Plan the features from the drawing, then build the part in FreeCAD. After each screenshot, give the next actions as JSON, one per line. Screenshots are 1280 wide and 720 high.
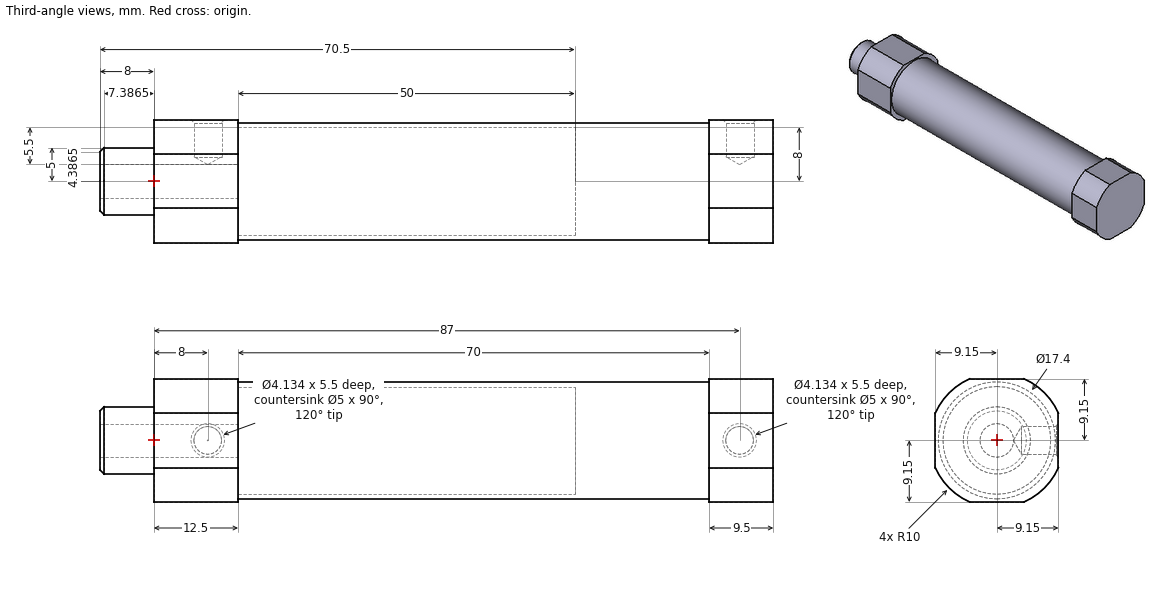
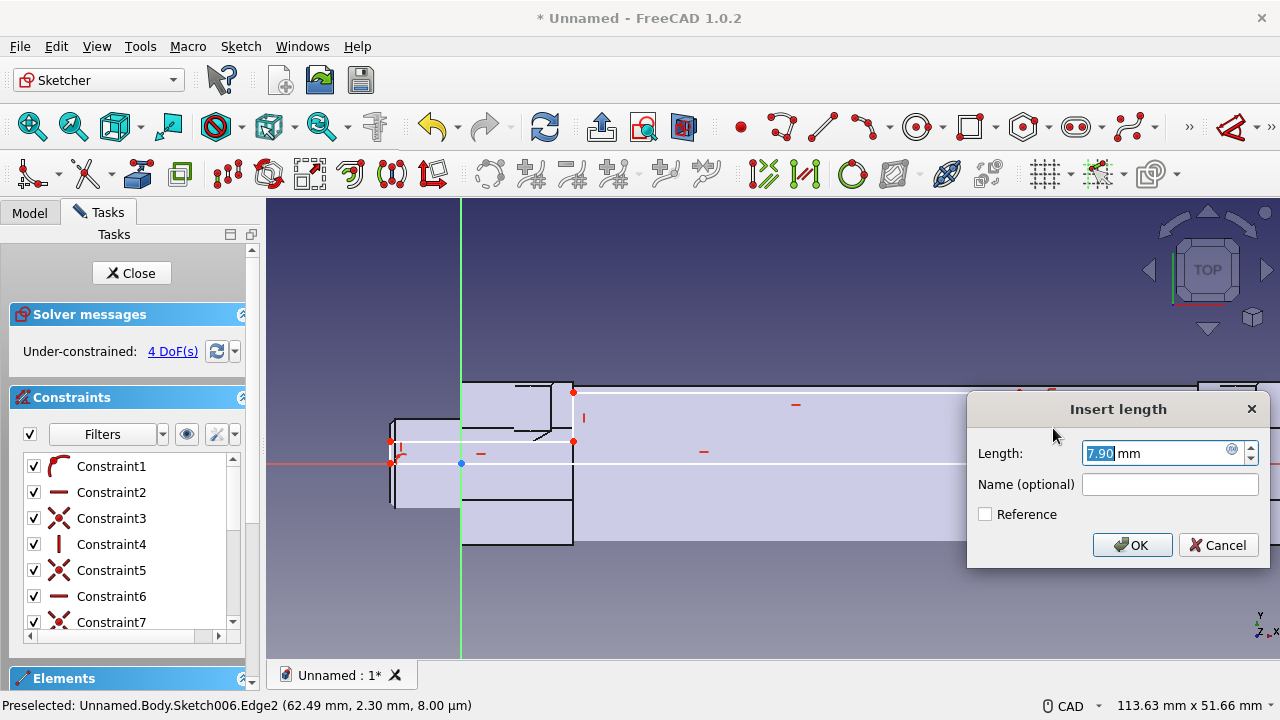
{"action": "type", "text": "8"}
{"action": "key", "text": "Return"}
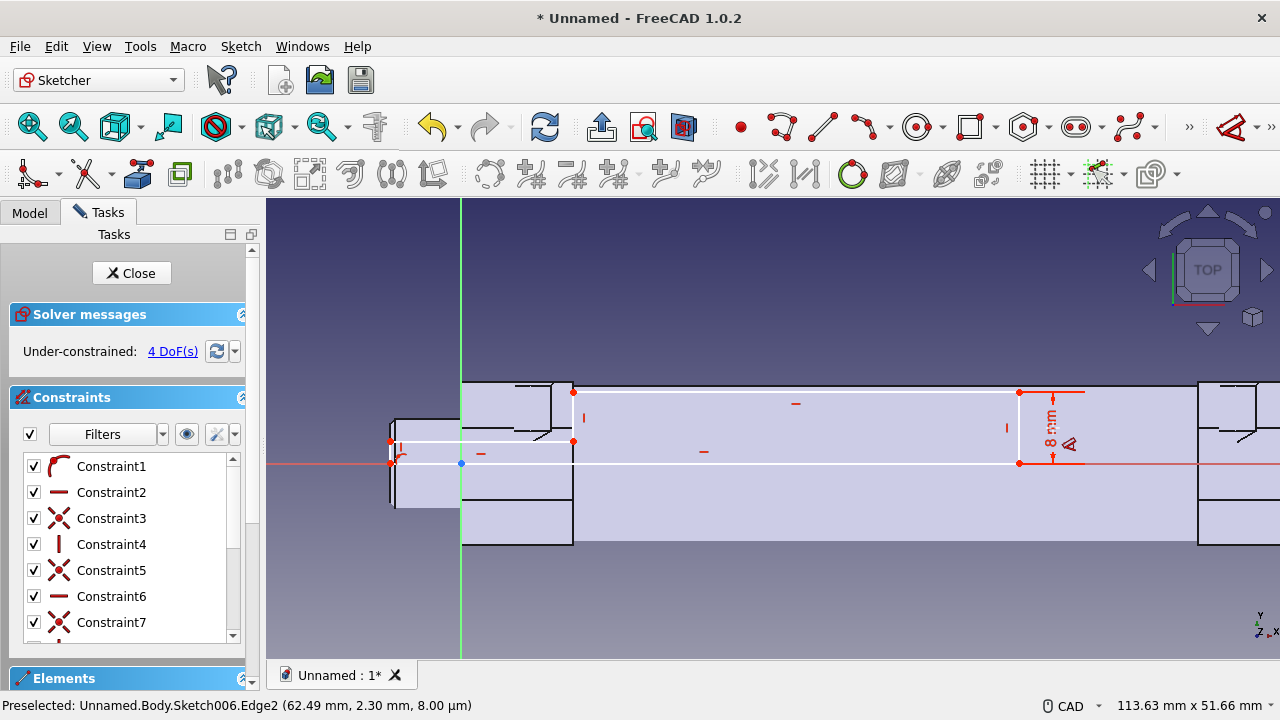
{"action": "left_click", "coordinate": [885, 392]}
{"action": "left_click", "coordinate": [796, 358]}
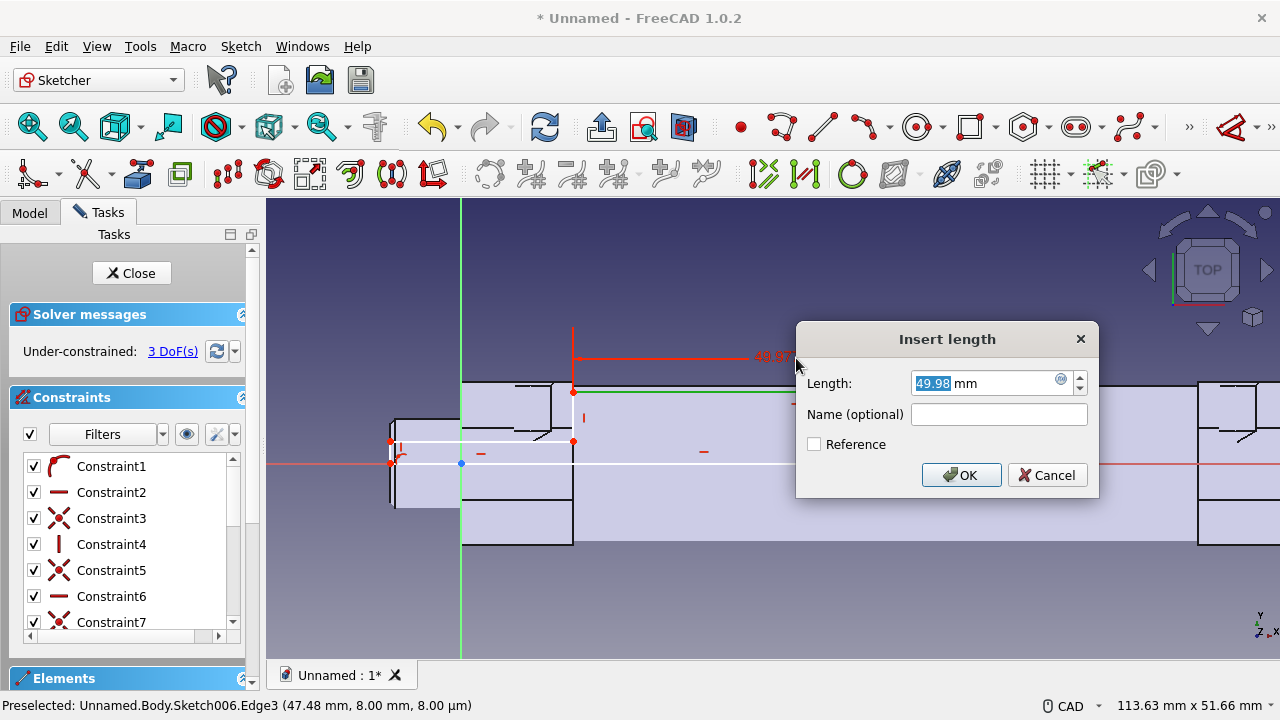
{"action": "type", "text": "50"}
{"action": "key", "text": "Return"}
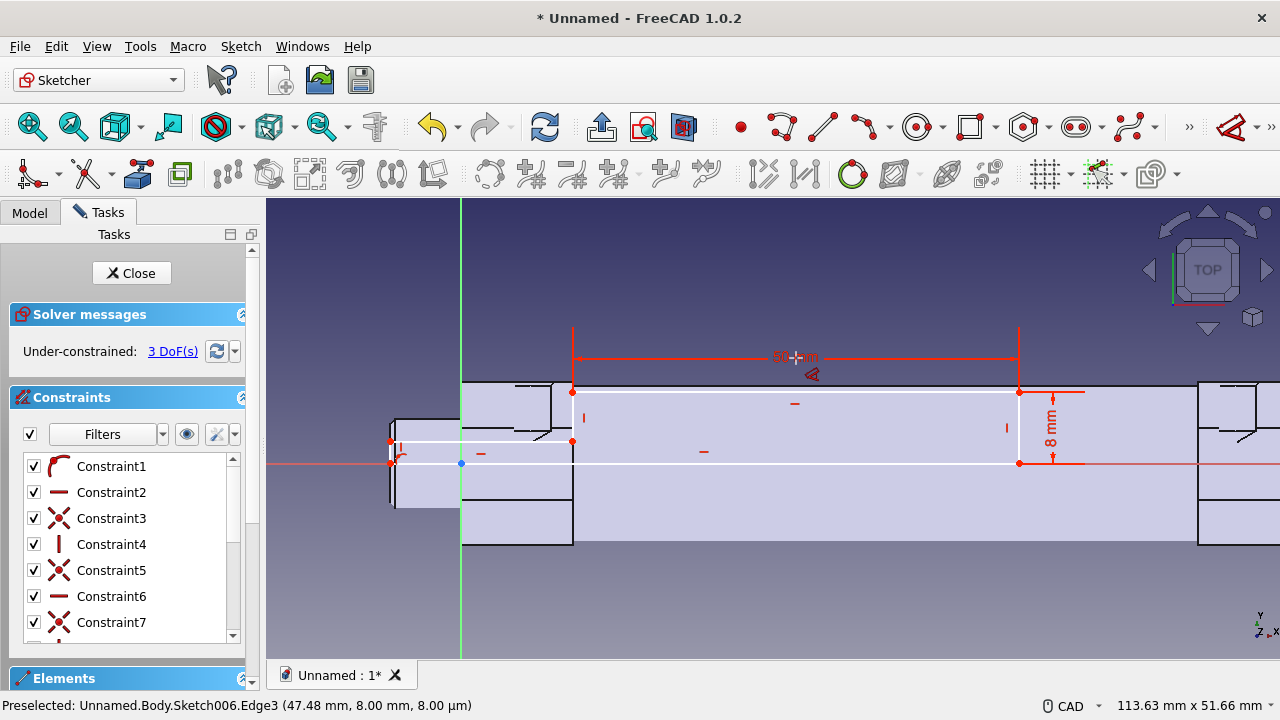
{"action": "left_click", "coordinate": [390, 464]}
{"action": "left_click", "coordinate": [426, 498]}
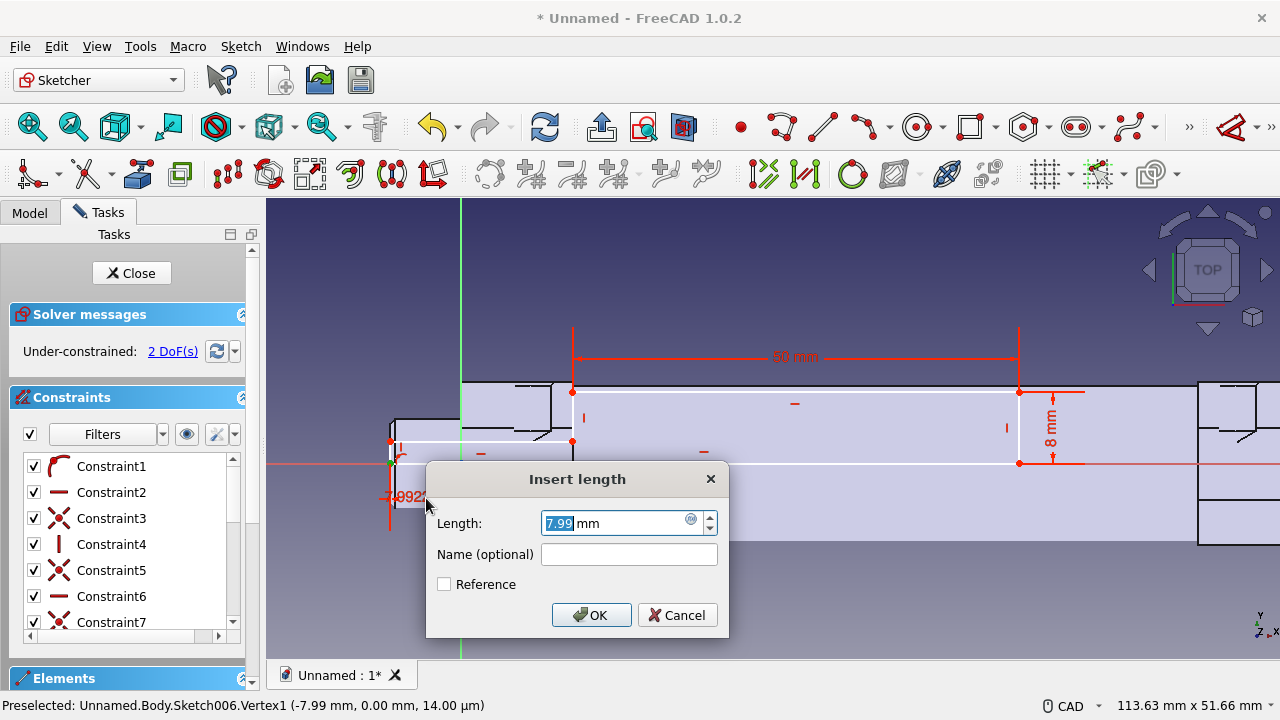
{"action": "type", "text": "8"}
{"action": "key", "text": "Return"}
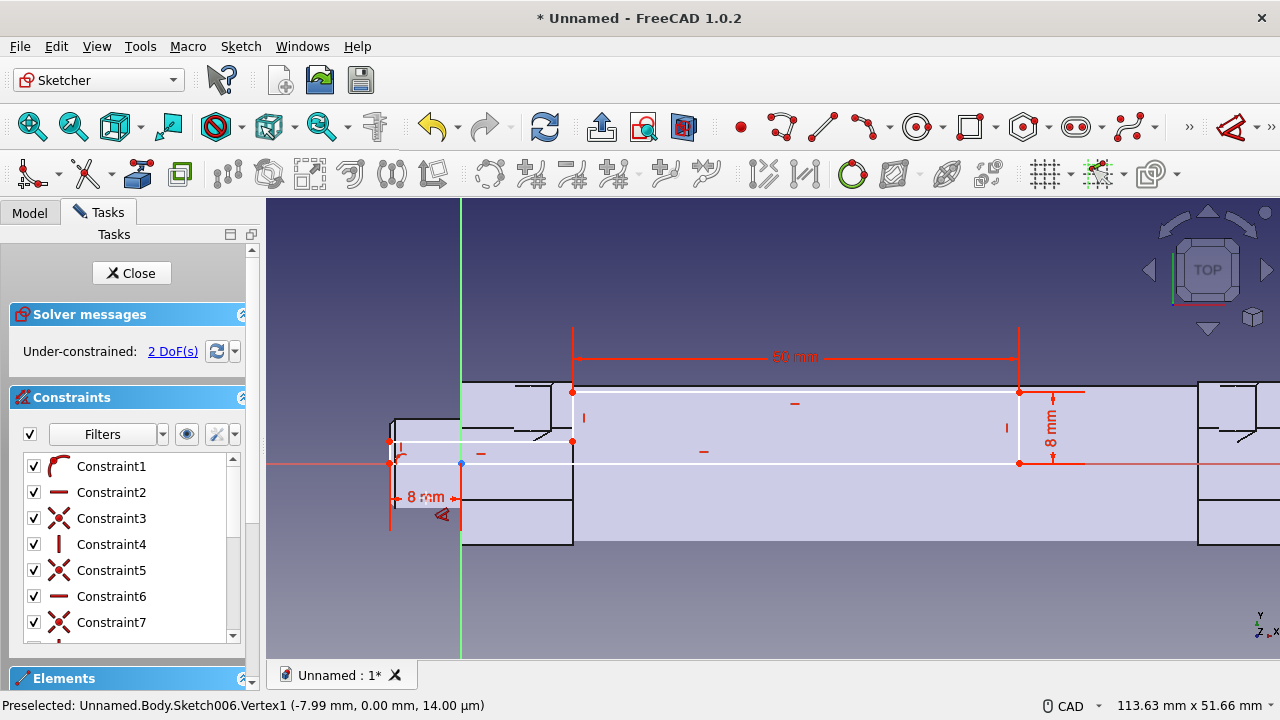
{"action": "left_click", "coordinate": [573, 407]}
{"action": "left_click", "coordinate": [539, 417]}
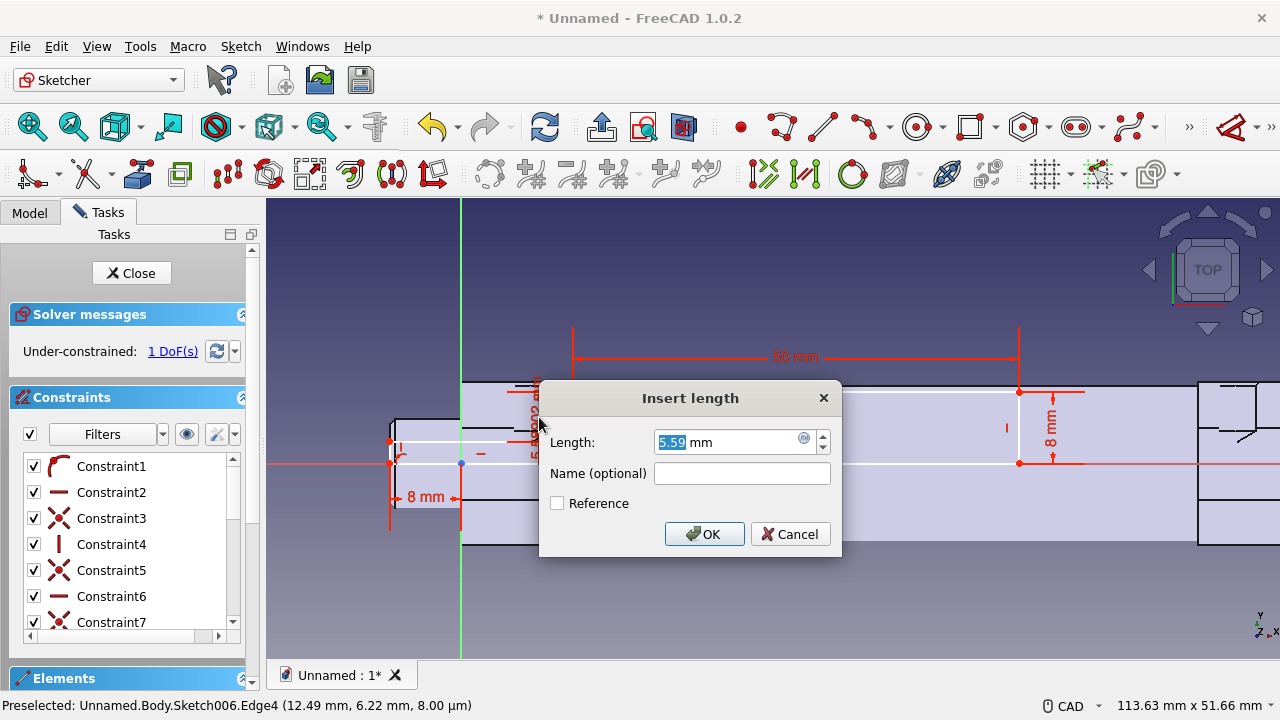
{"action": "type", "text": "5.5"}
{"action": "key", "text": "Return"}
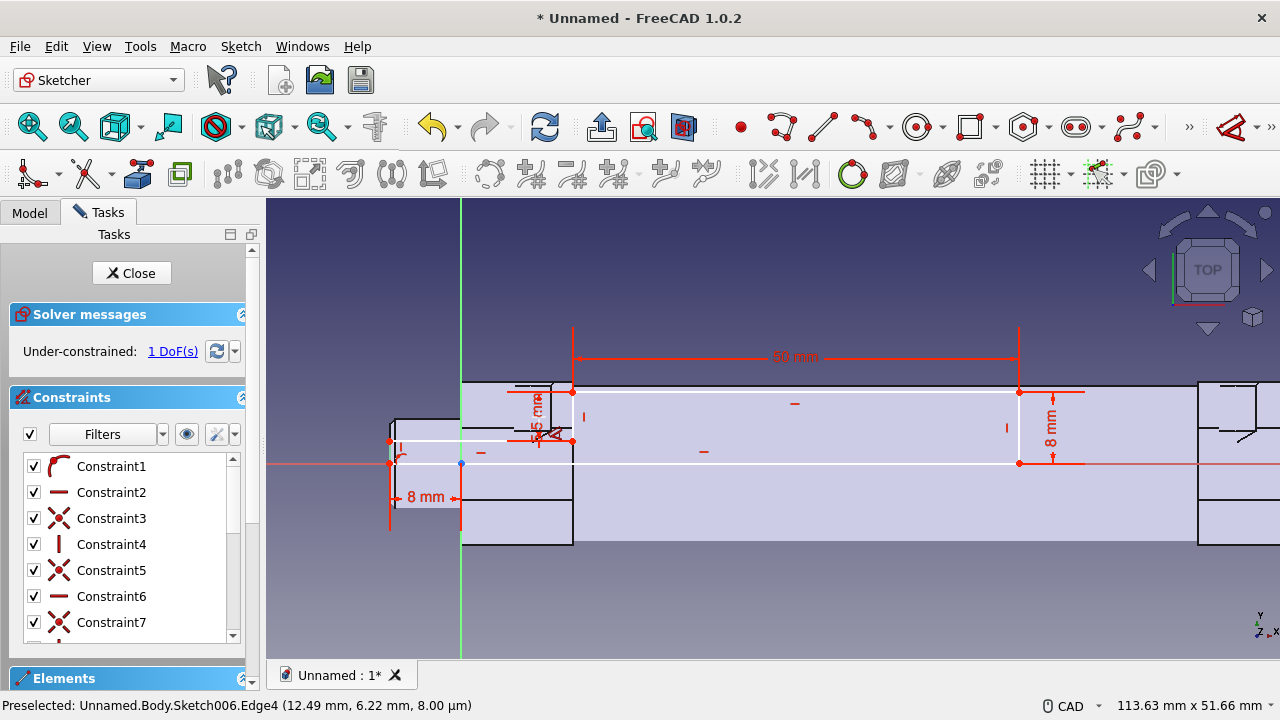
{"action": "left_click", "coordinate": [579, 464]}
{"action": "left_click", "coordinate": [704, 498]}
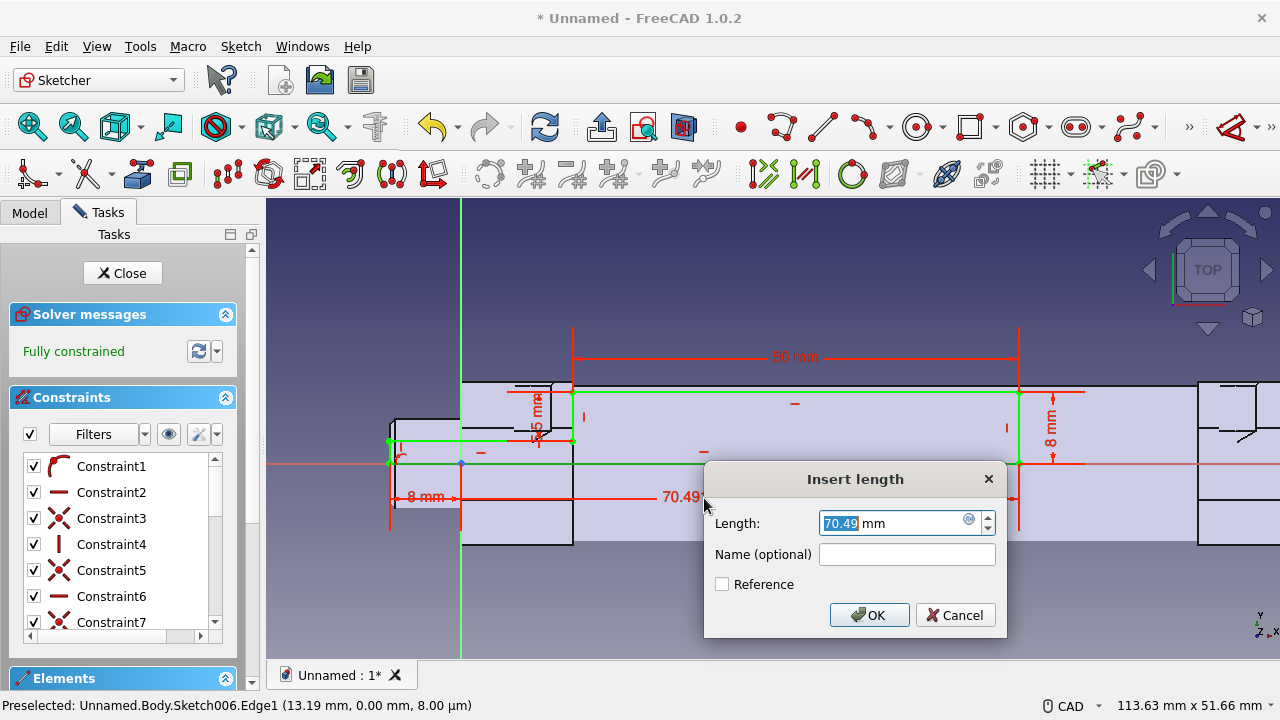
{"action": "type", "text": "70.5"}
{"action": "key", "text": "Return"}
{"action": "key", "text": "Escape"}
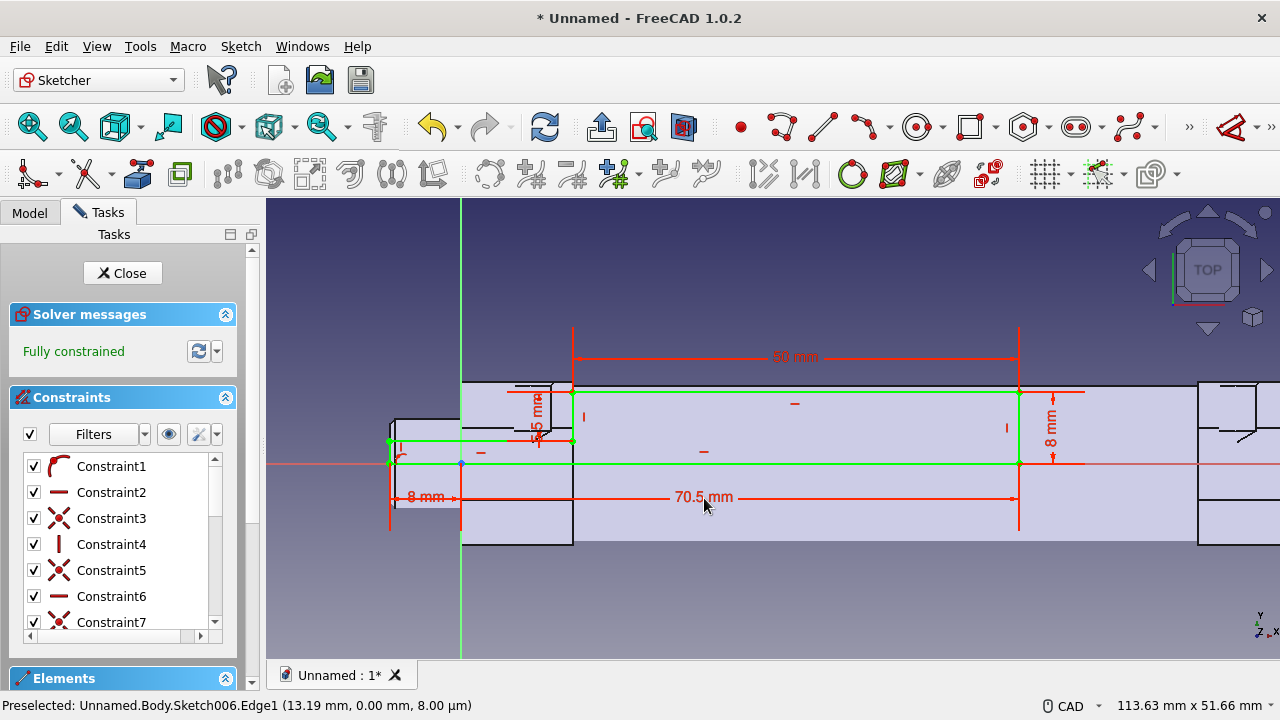
{"action": "left_click", "coordinate": [123, 273]}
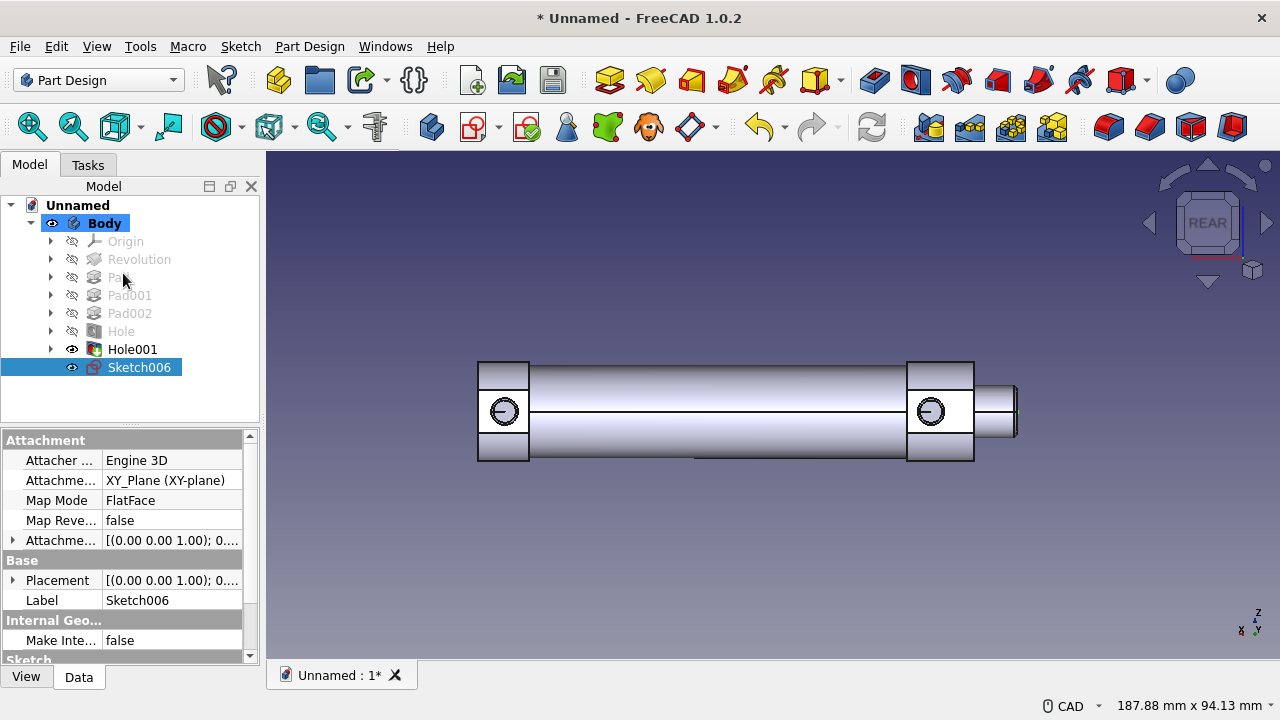
{"action": "left_click", "coordinate": [957, 80]}